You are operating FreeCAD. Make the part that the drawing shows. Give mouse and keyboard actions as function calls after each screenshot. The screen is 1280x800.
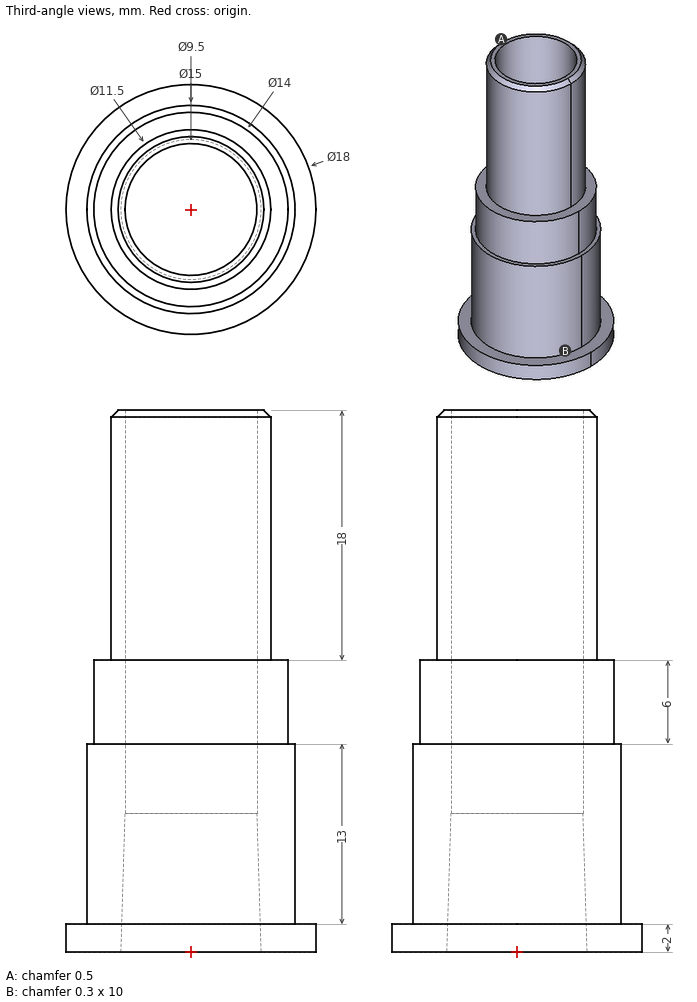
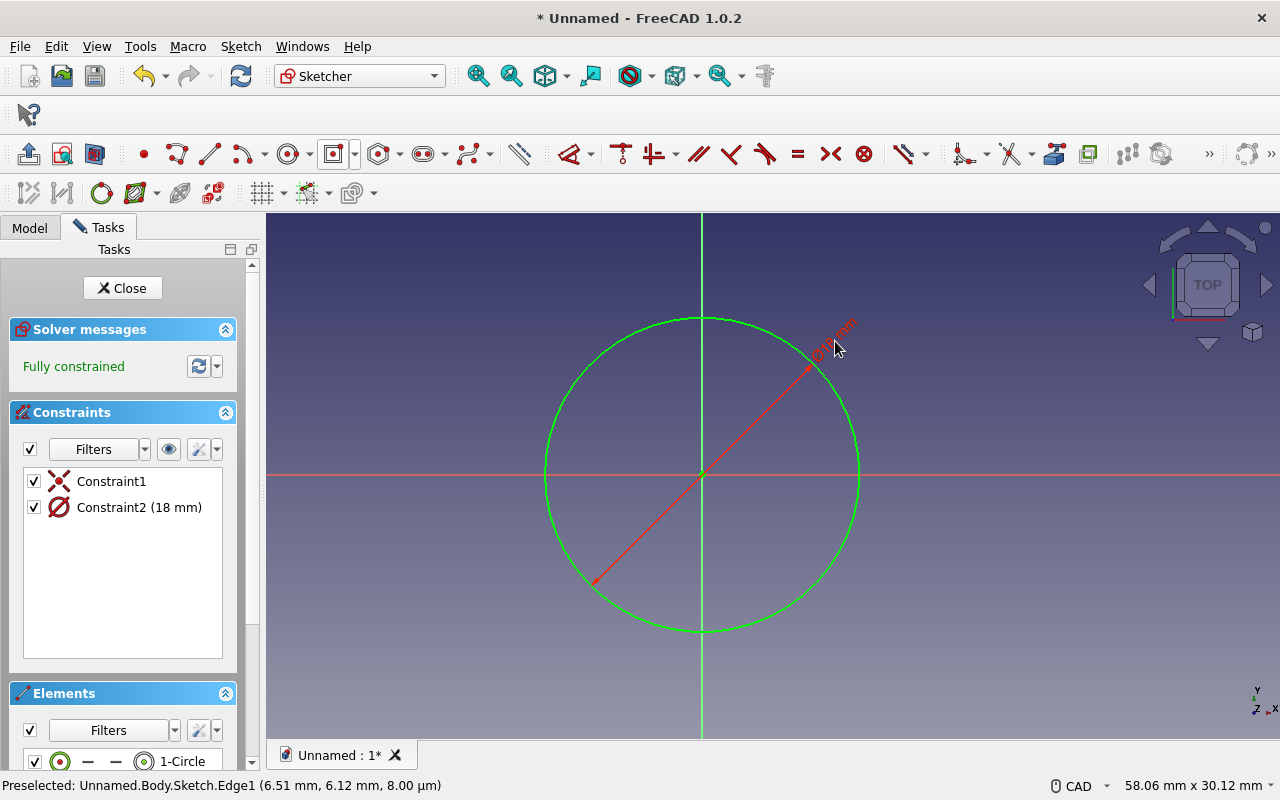
click(123, 288)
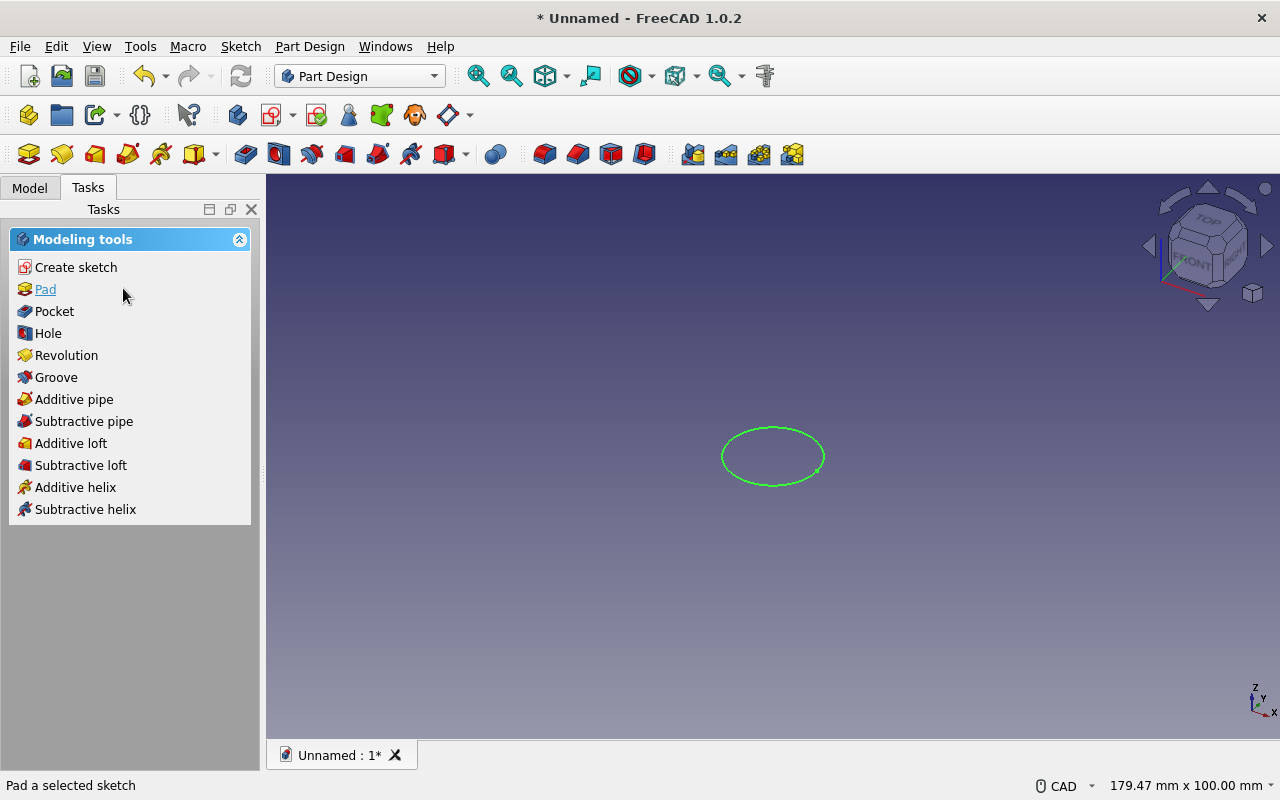
click(29, 154)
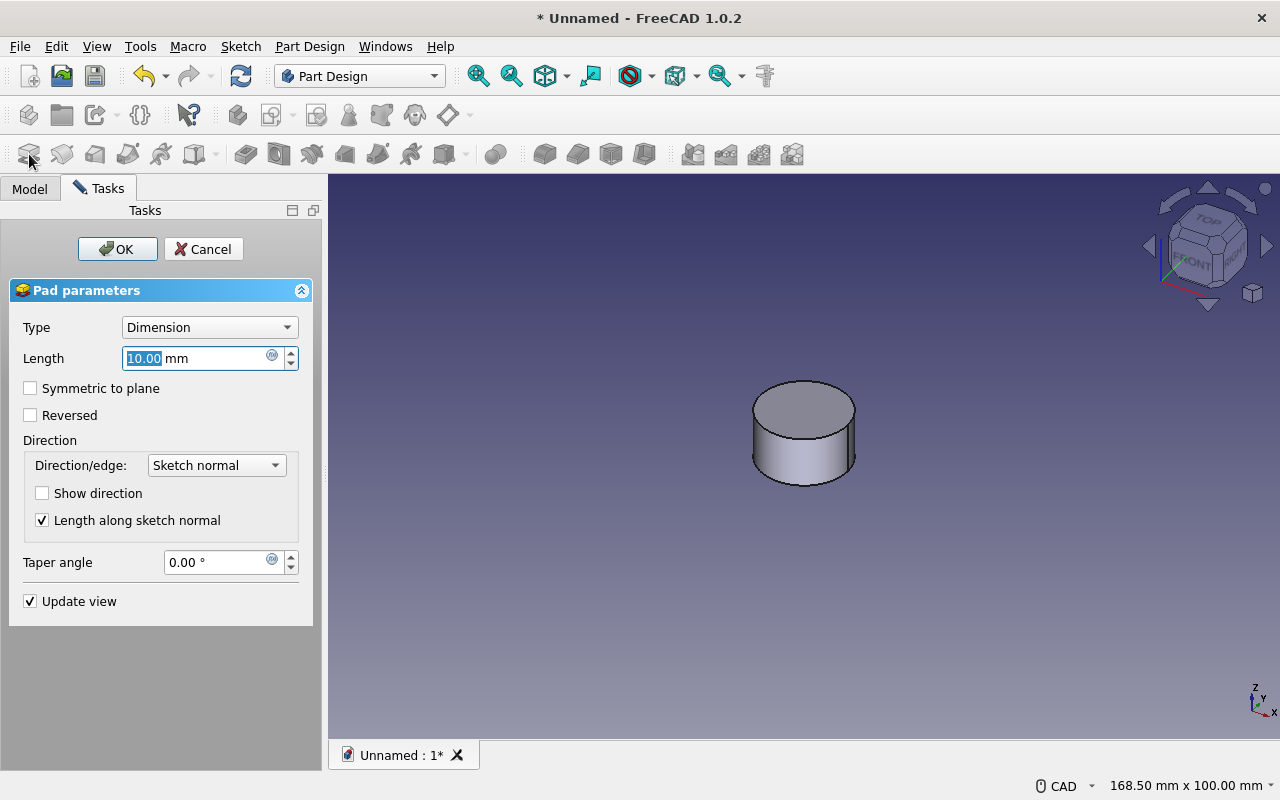
text(2)
key(Tab)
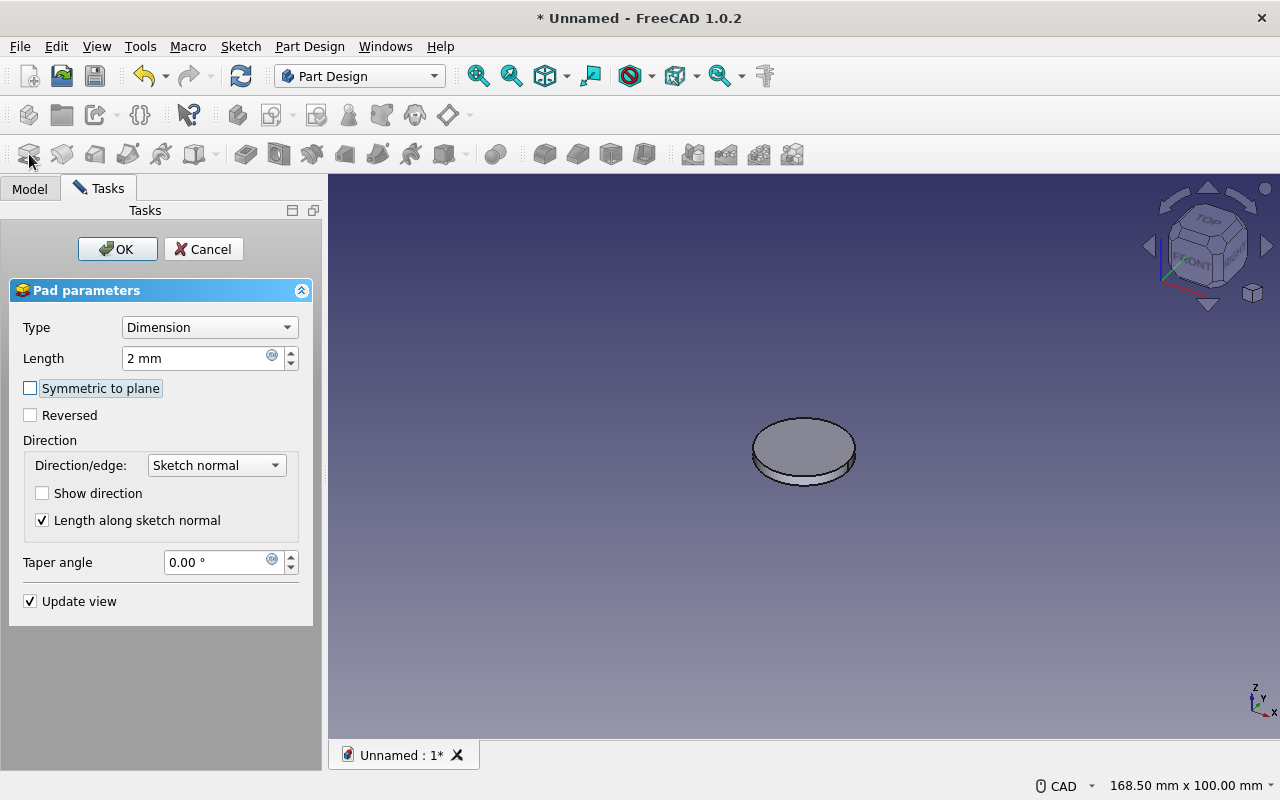
click(118, 249)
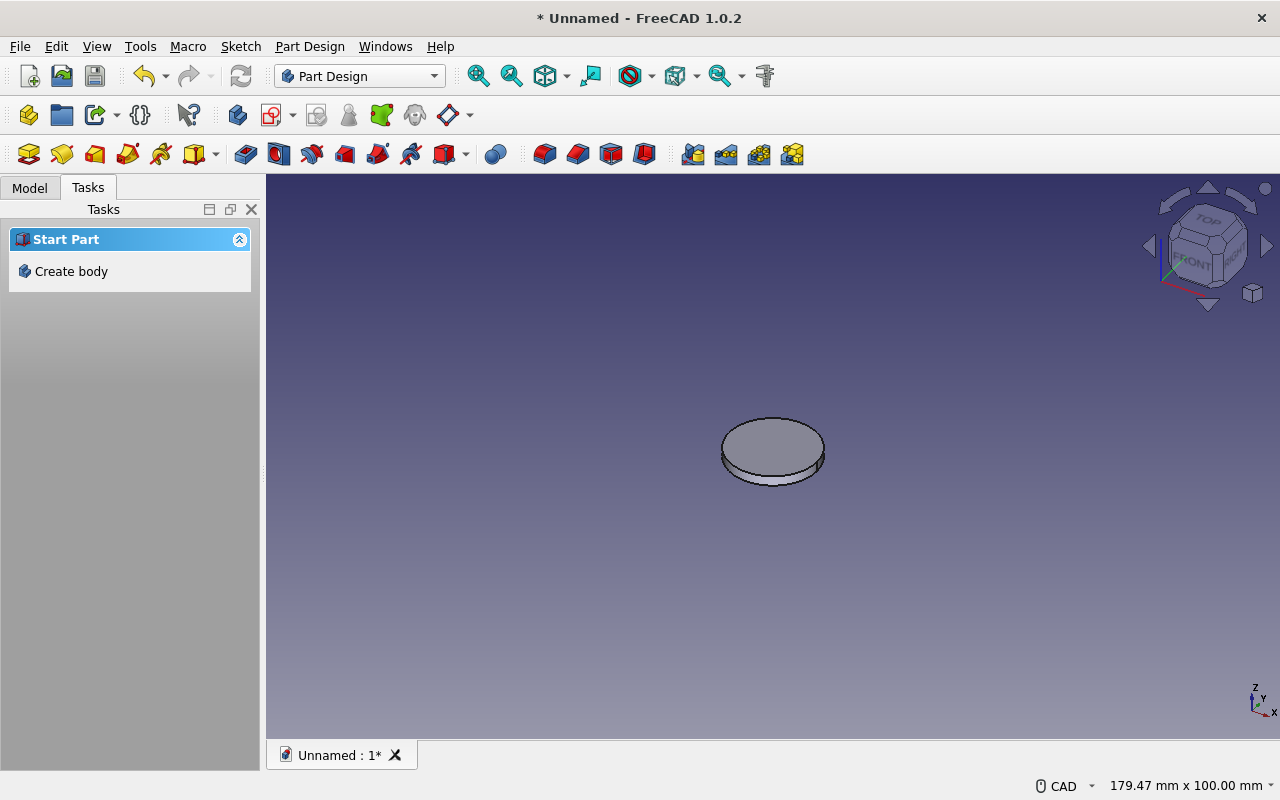
click(479, 76)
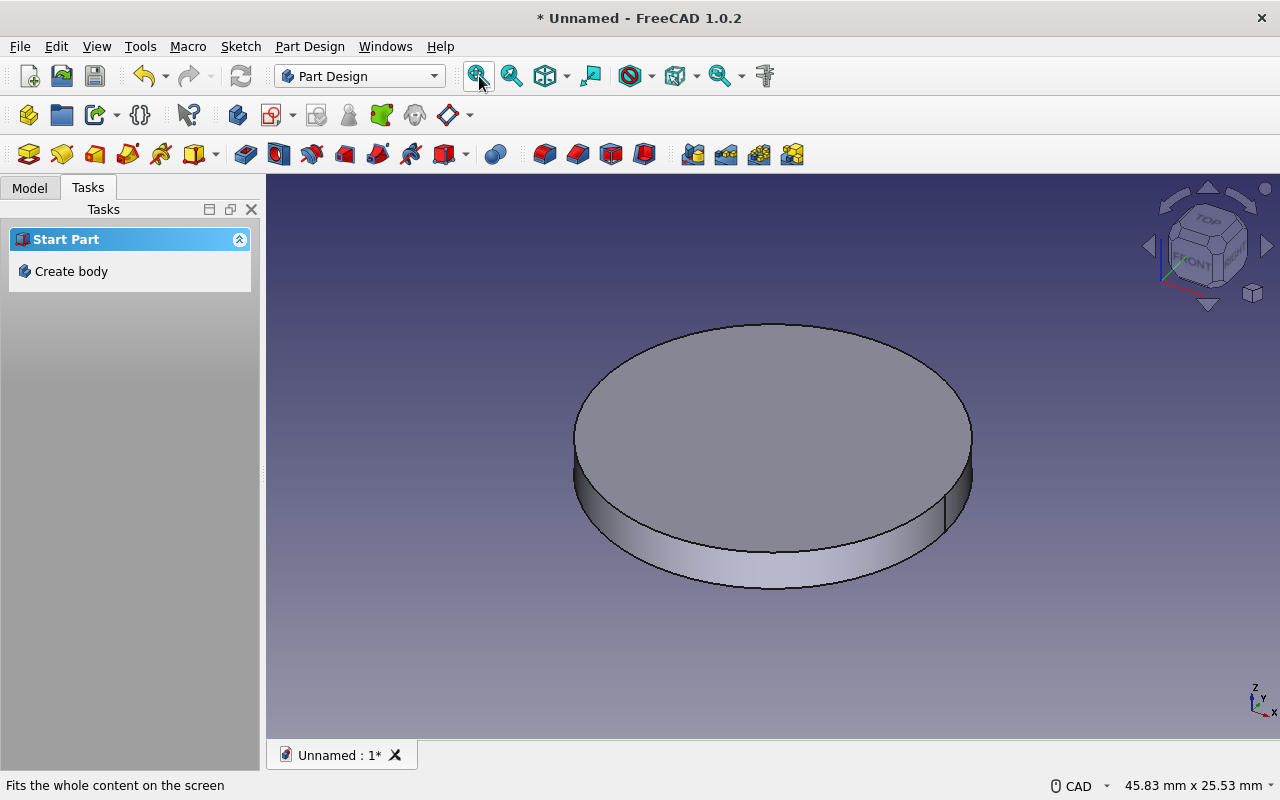
click(773, 437)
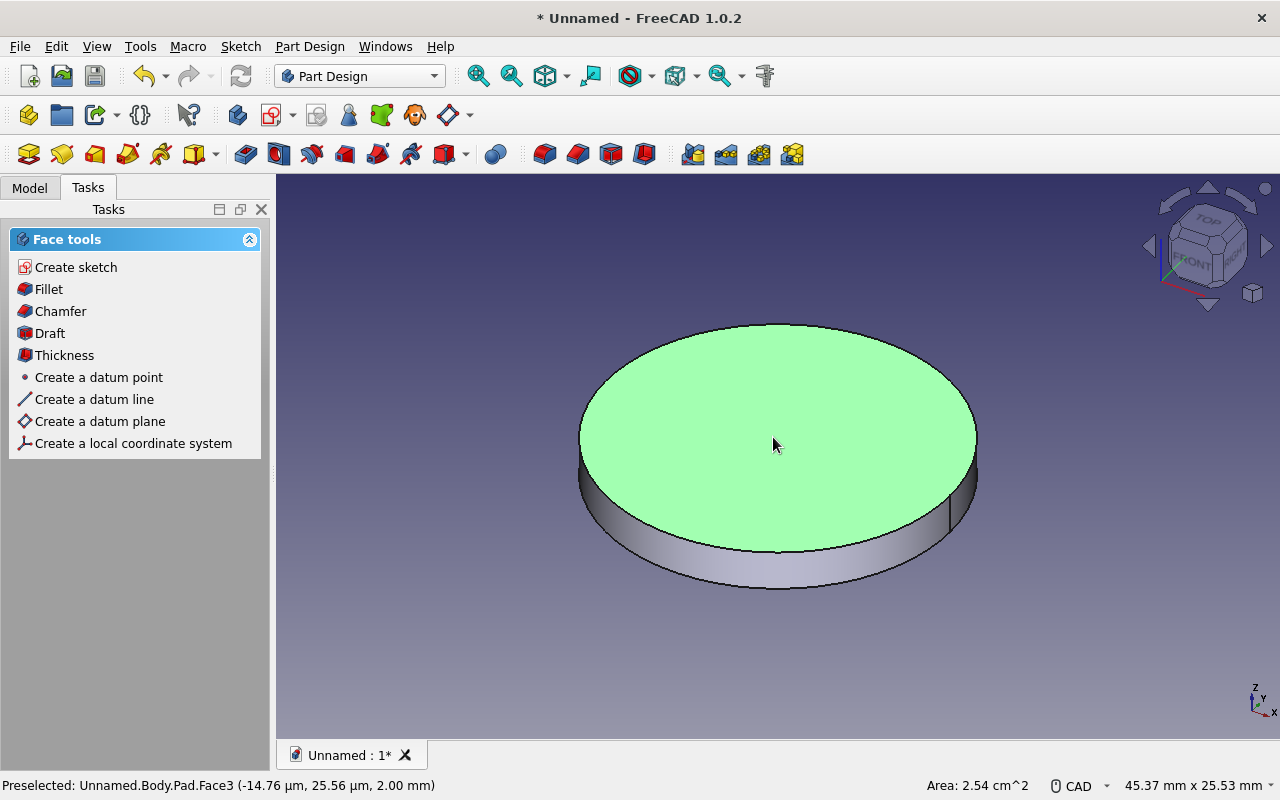
click(270, 116)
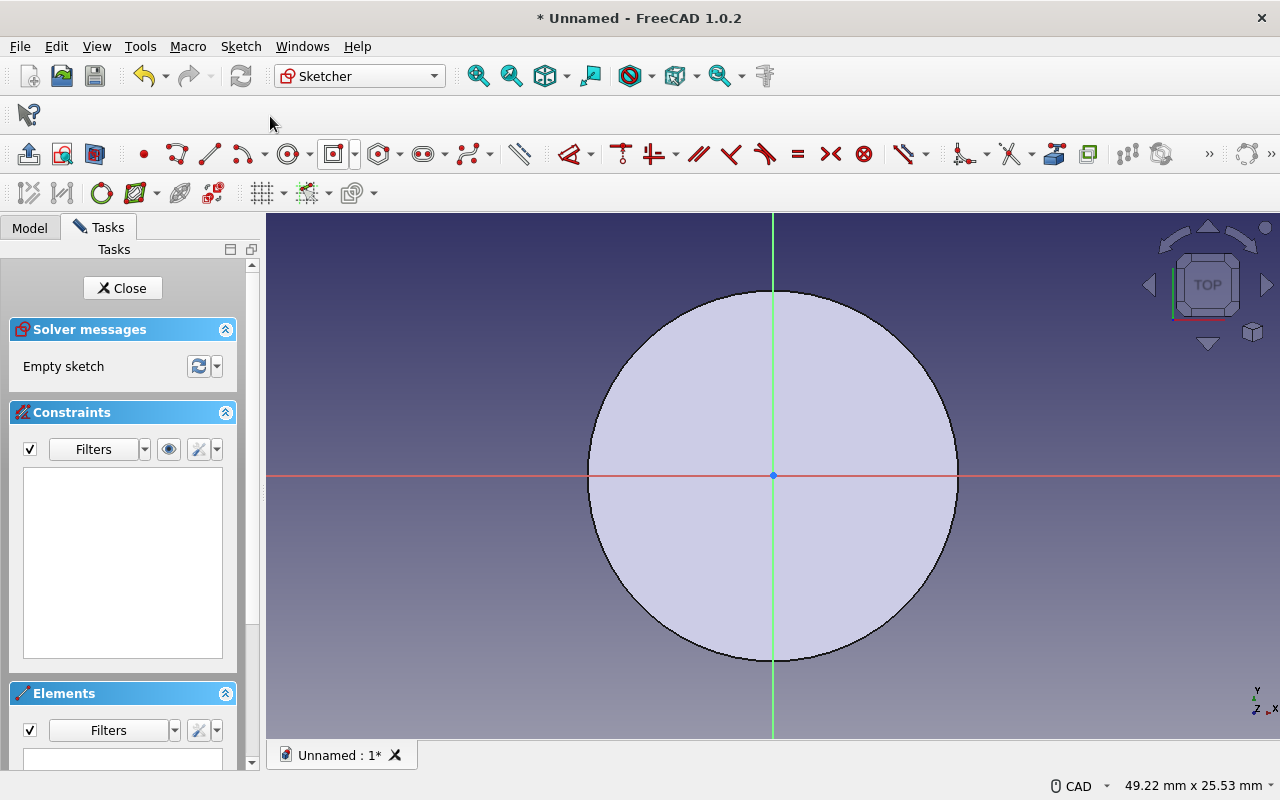
click(288, 154)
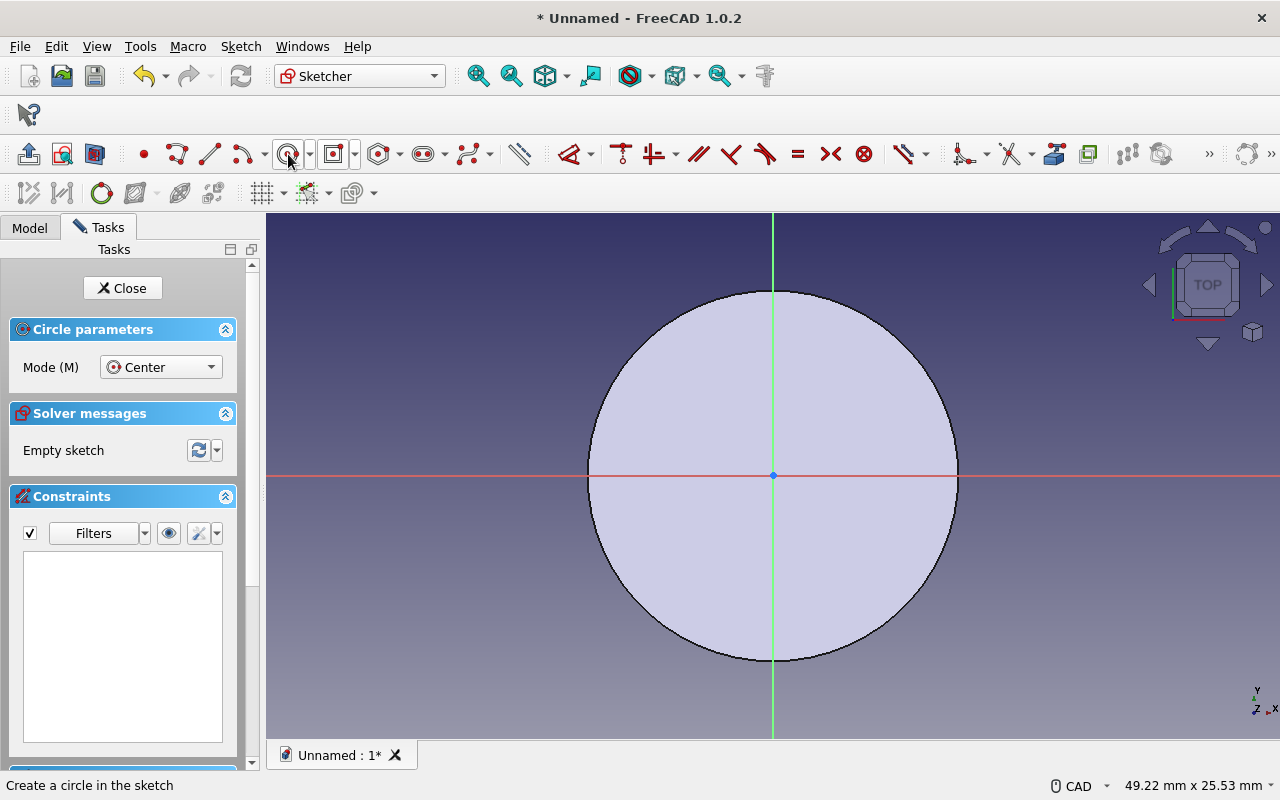
click(773, 476)
click(882, 367)
key(Escape)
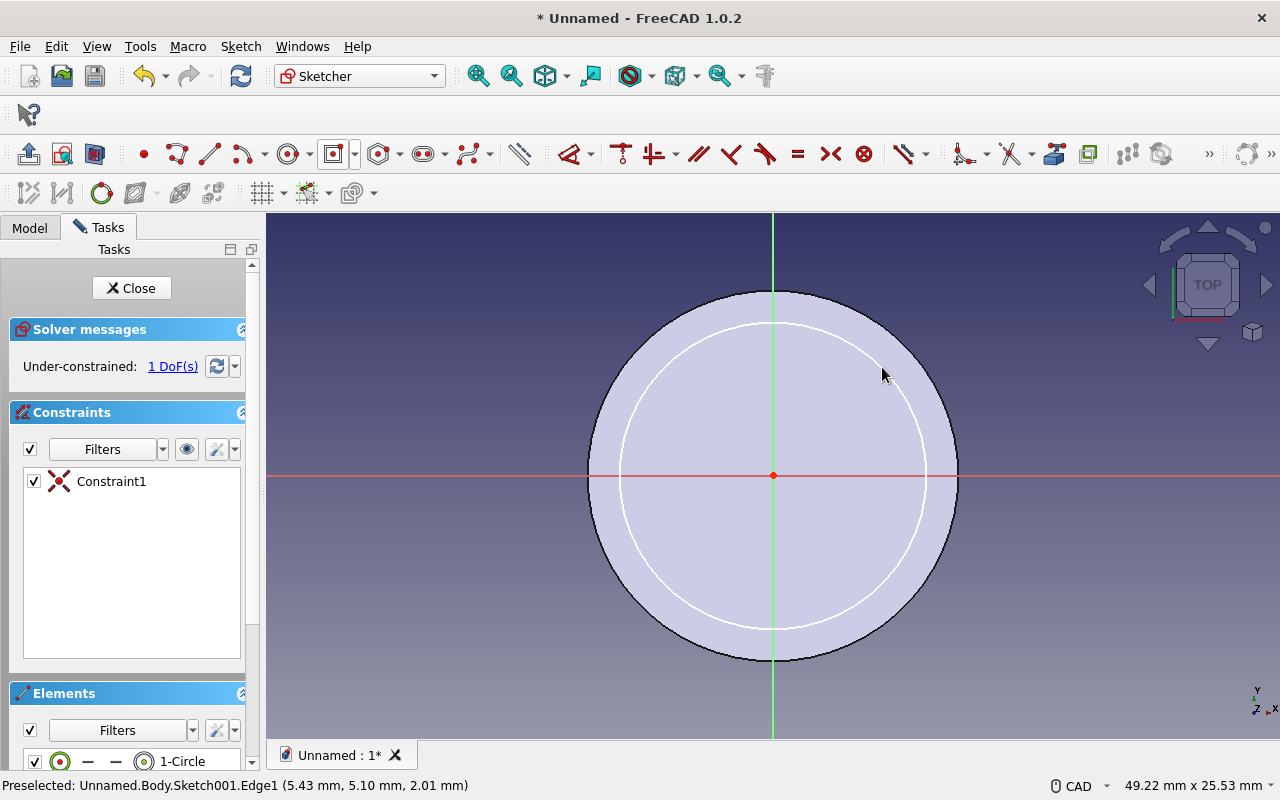
click(568, 154)